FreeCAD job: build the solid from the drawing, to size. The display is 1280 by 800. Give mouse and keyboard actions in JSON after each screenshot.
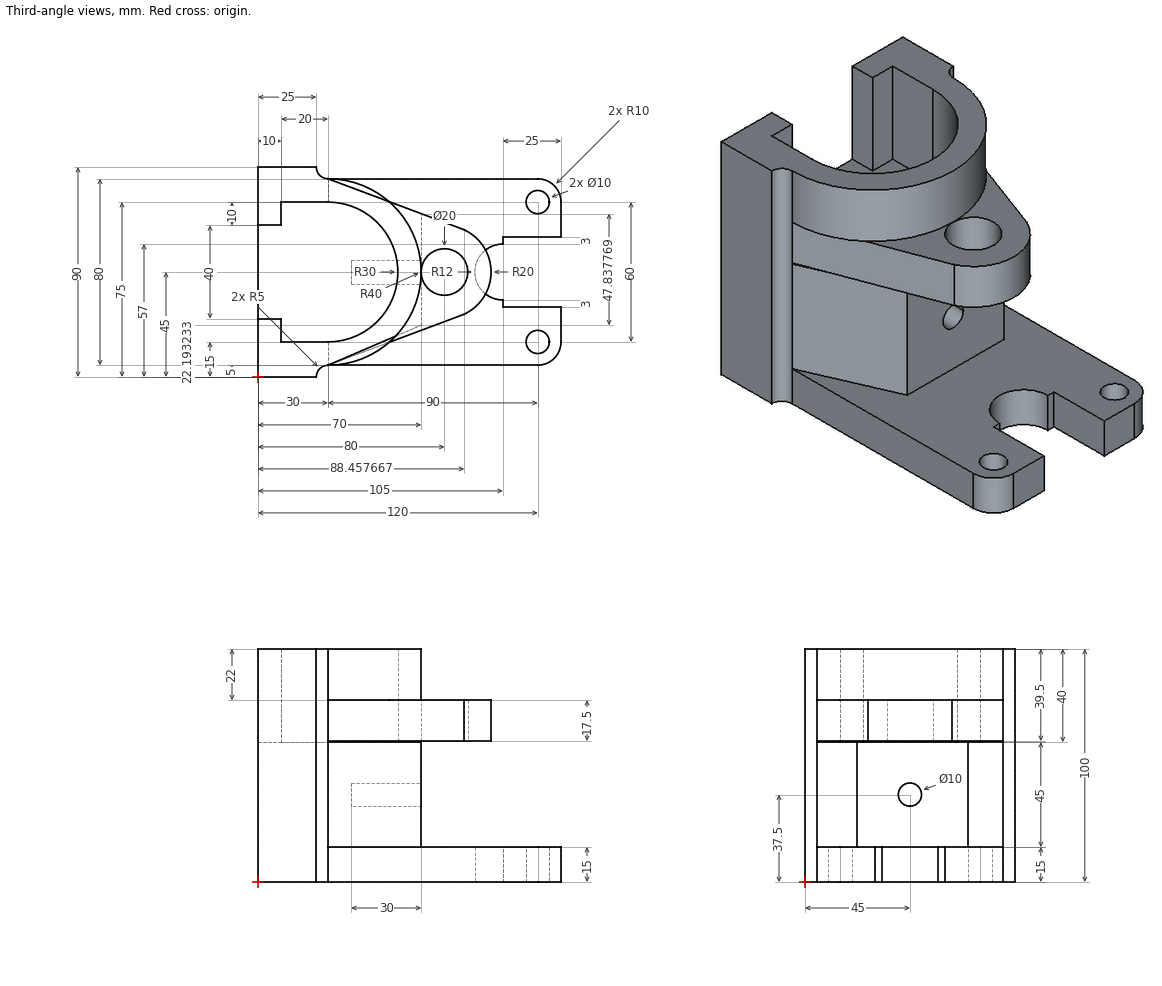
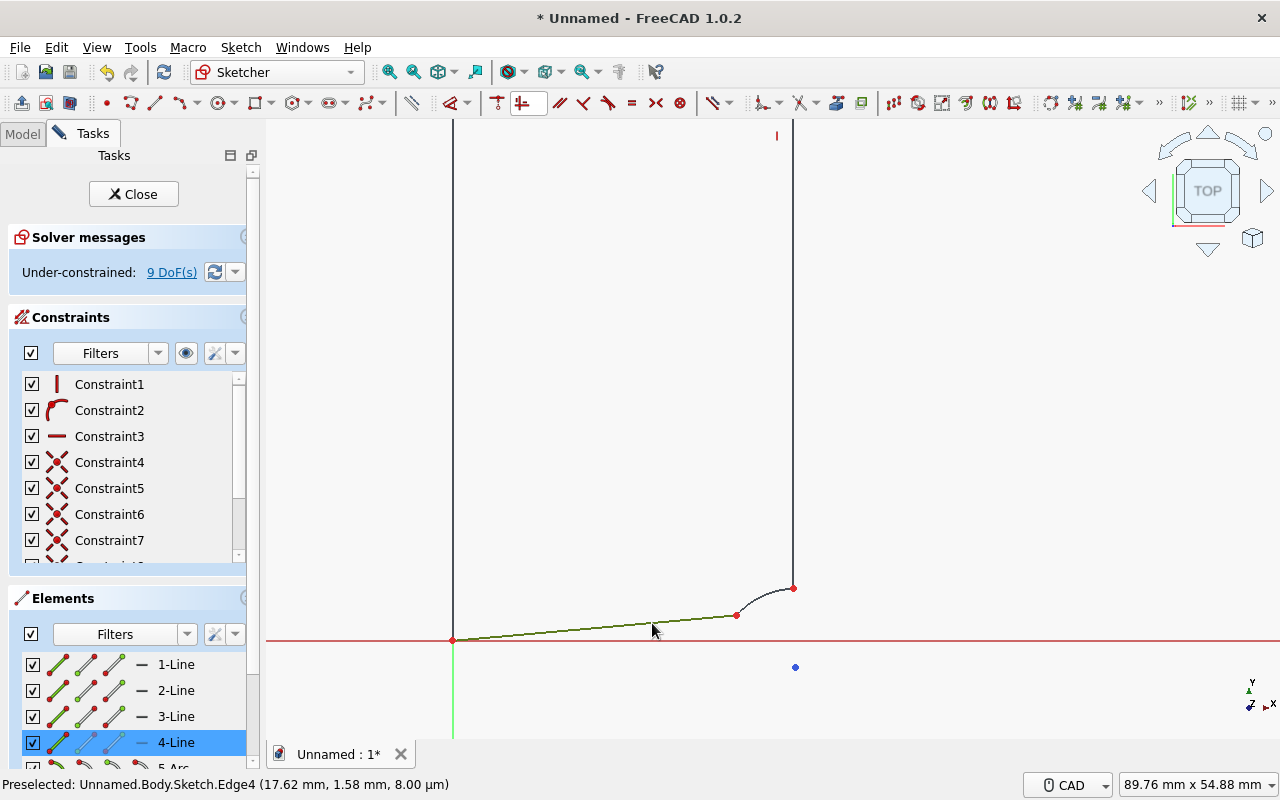
{"action": "left_click", "coordinate": [542, 104]}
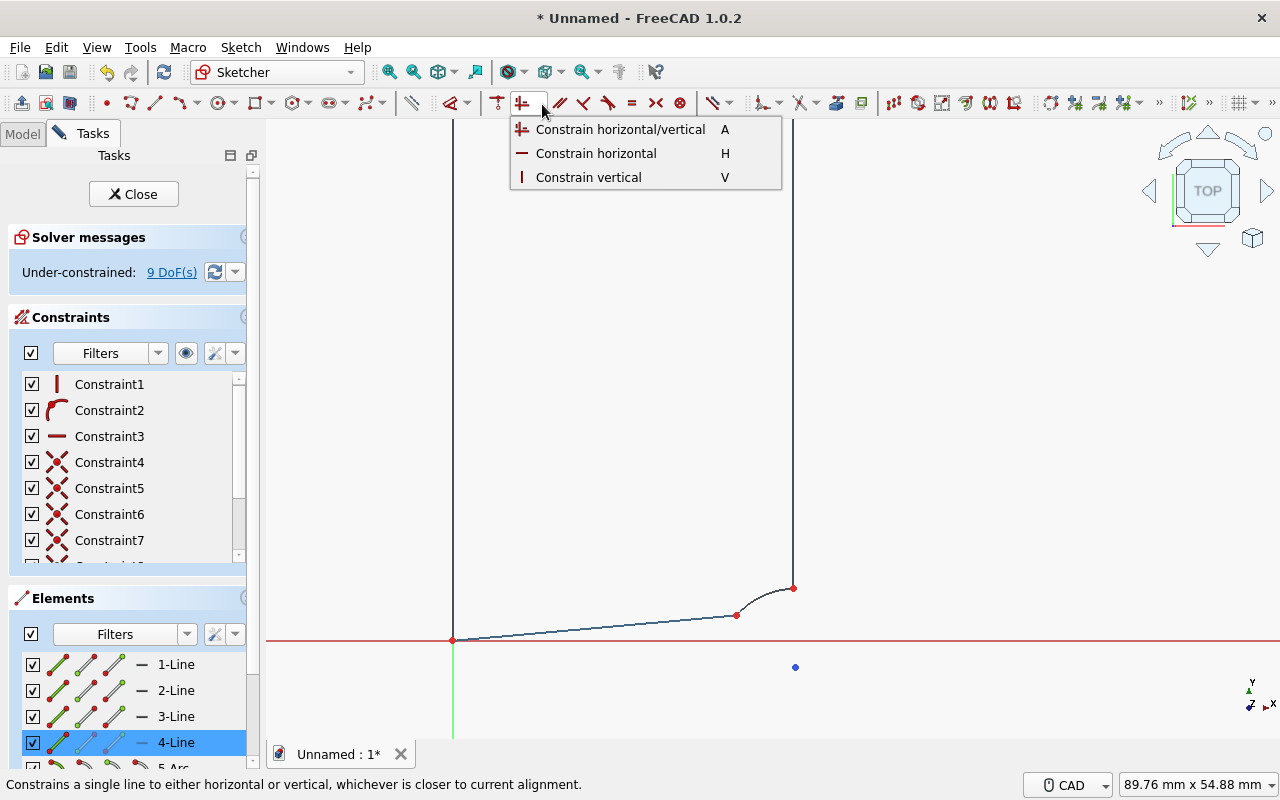
{"action": "left_click", "coordinate": [646, 153]}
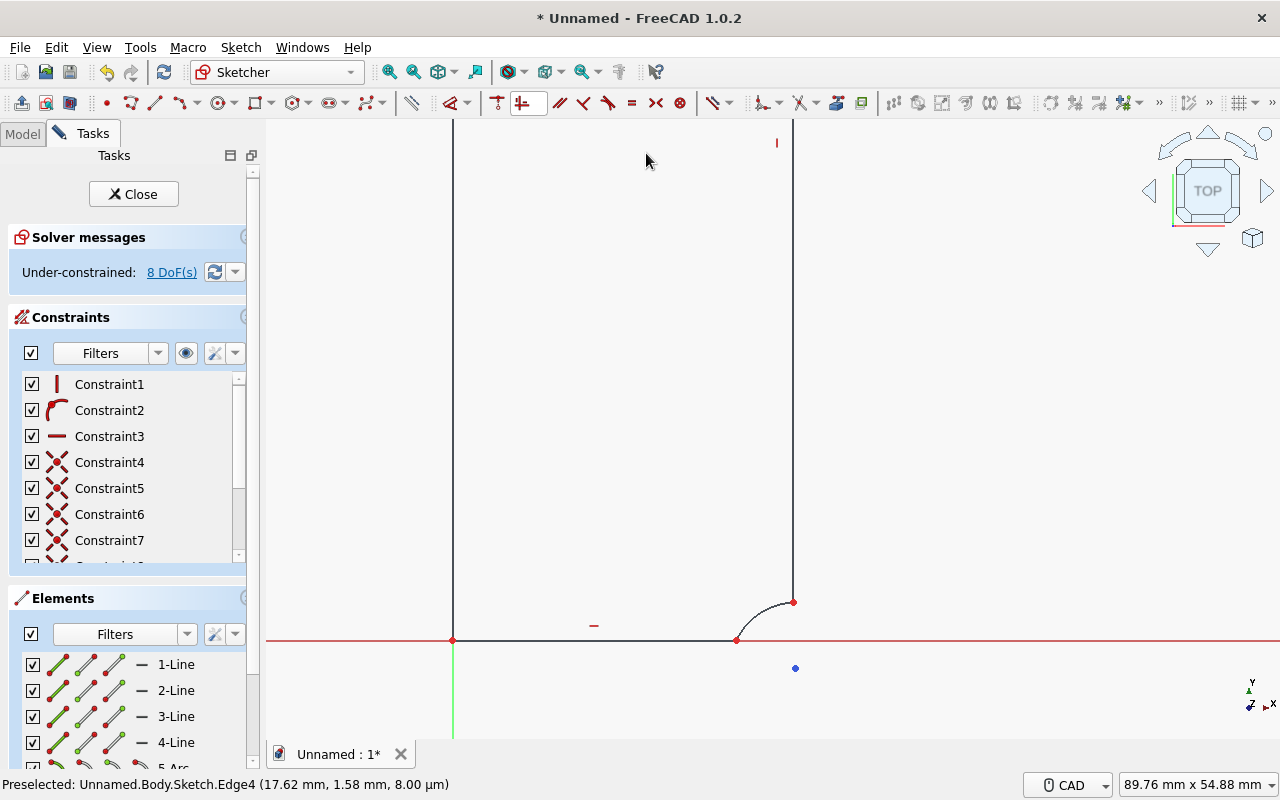
{"action": "scroll", "coordinate": [752, 602], "scroll_direction": "down", "scroll_amount": 5}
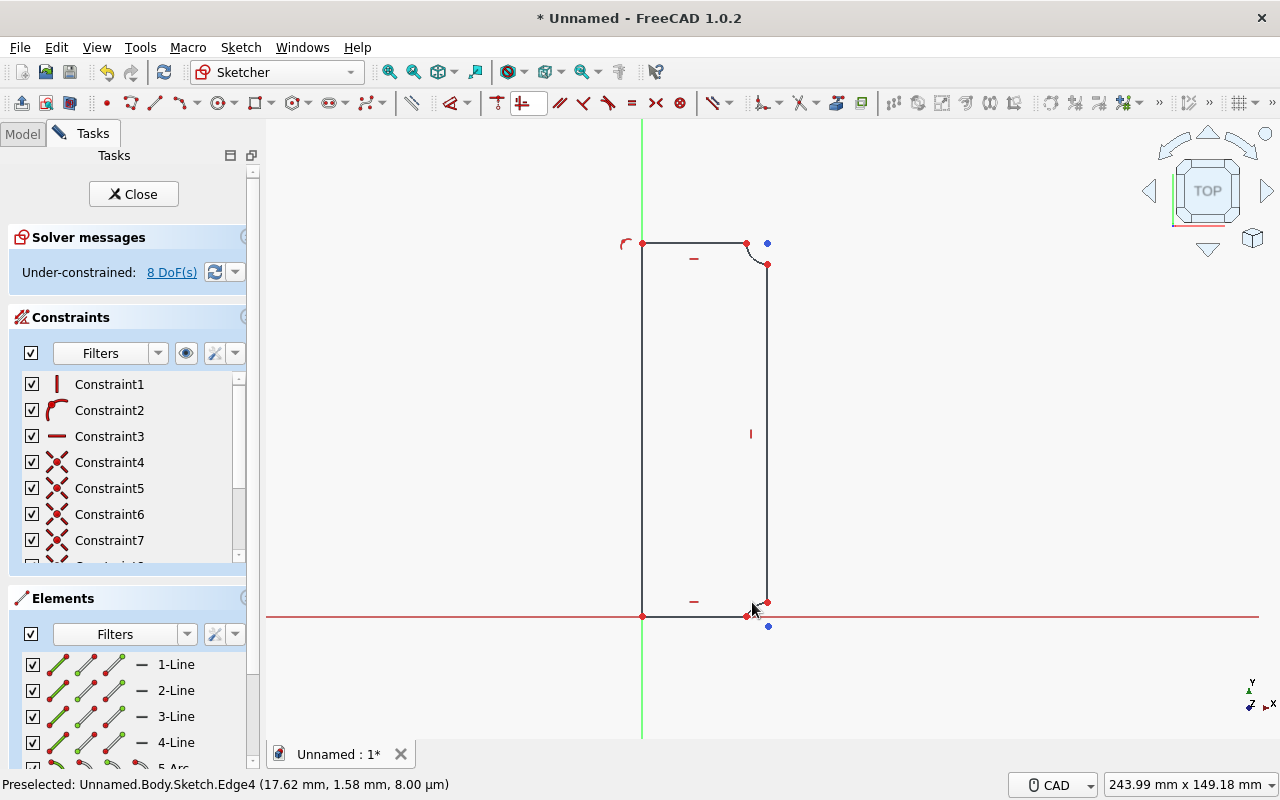
{"action": "scroll", "coordinate": [749, 253], "scroll_direction": "up", "scroll_amount": 2}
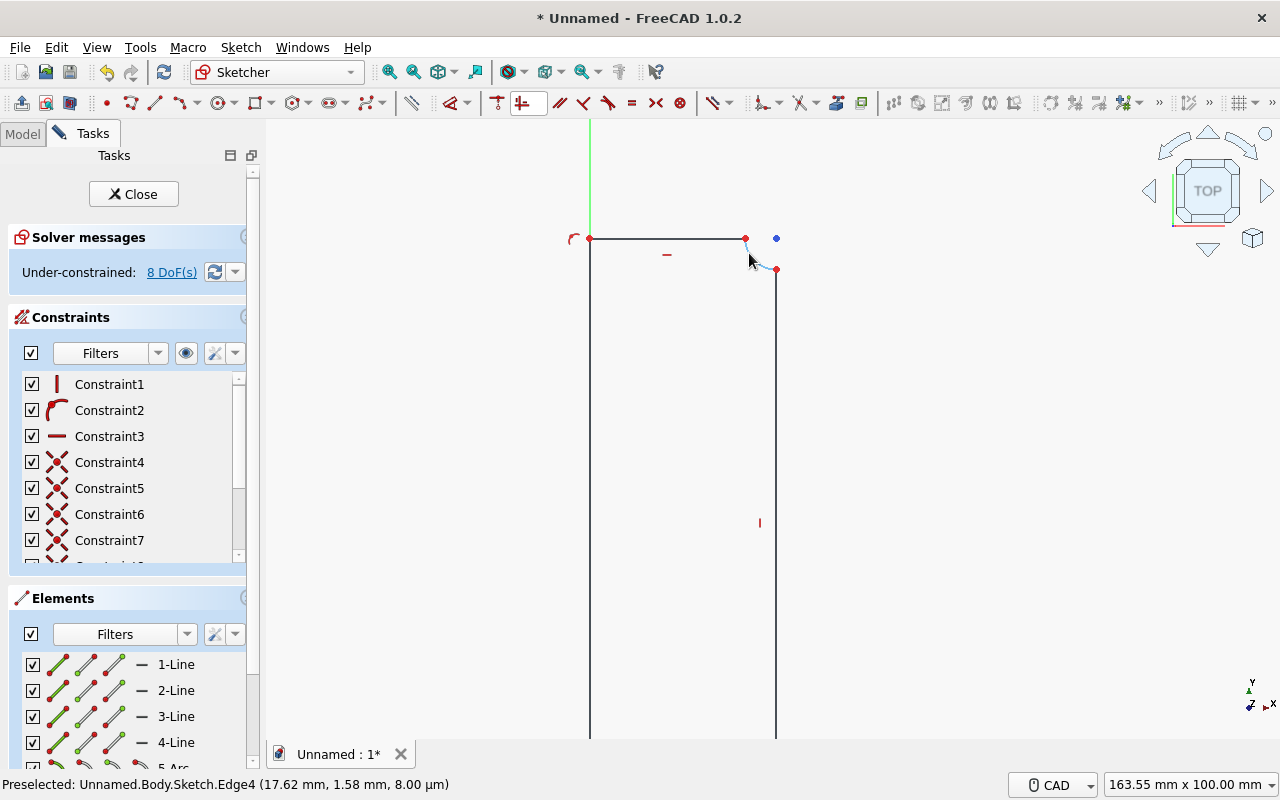
{"action": "left_click", "coordinate": [749, 253]}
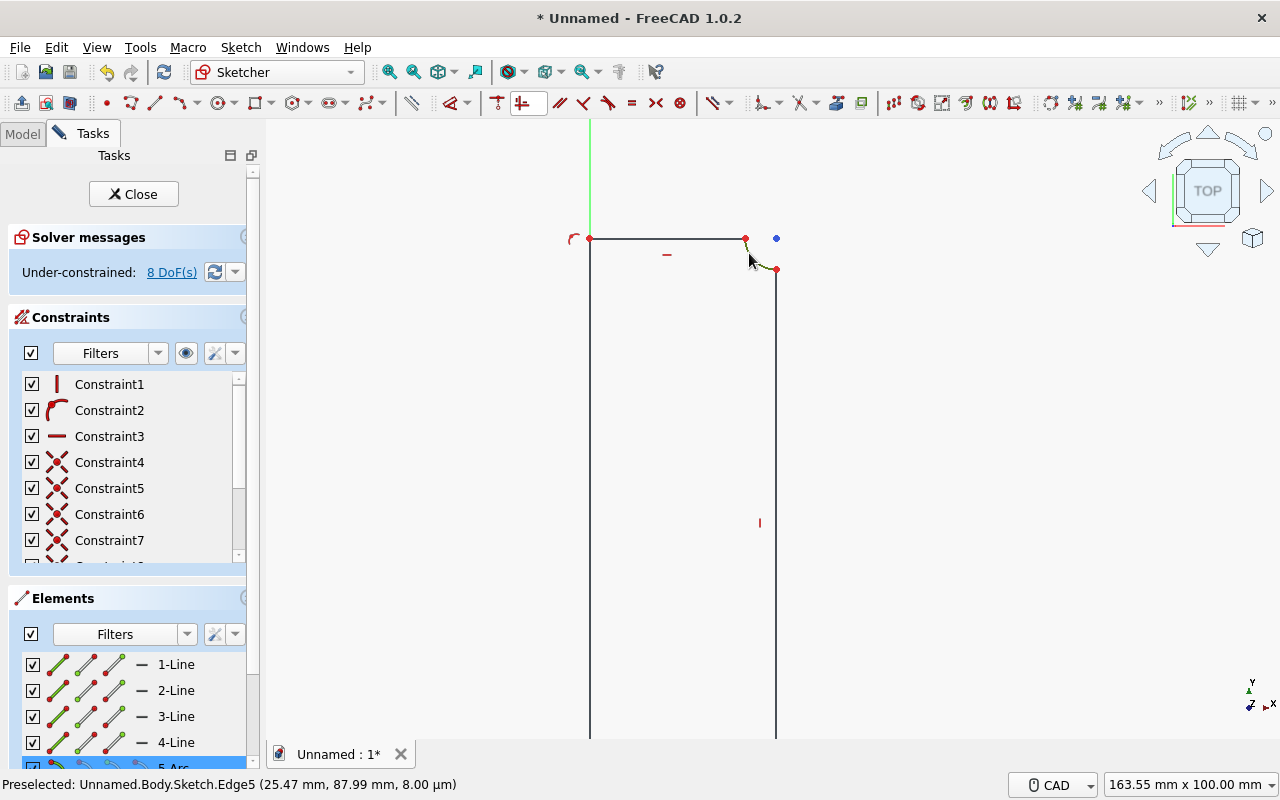
{"action": "scroll", "coordinate": [749, 251], "scroll_direction": "down", "scroll_amount": 2}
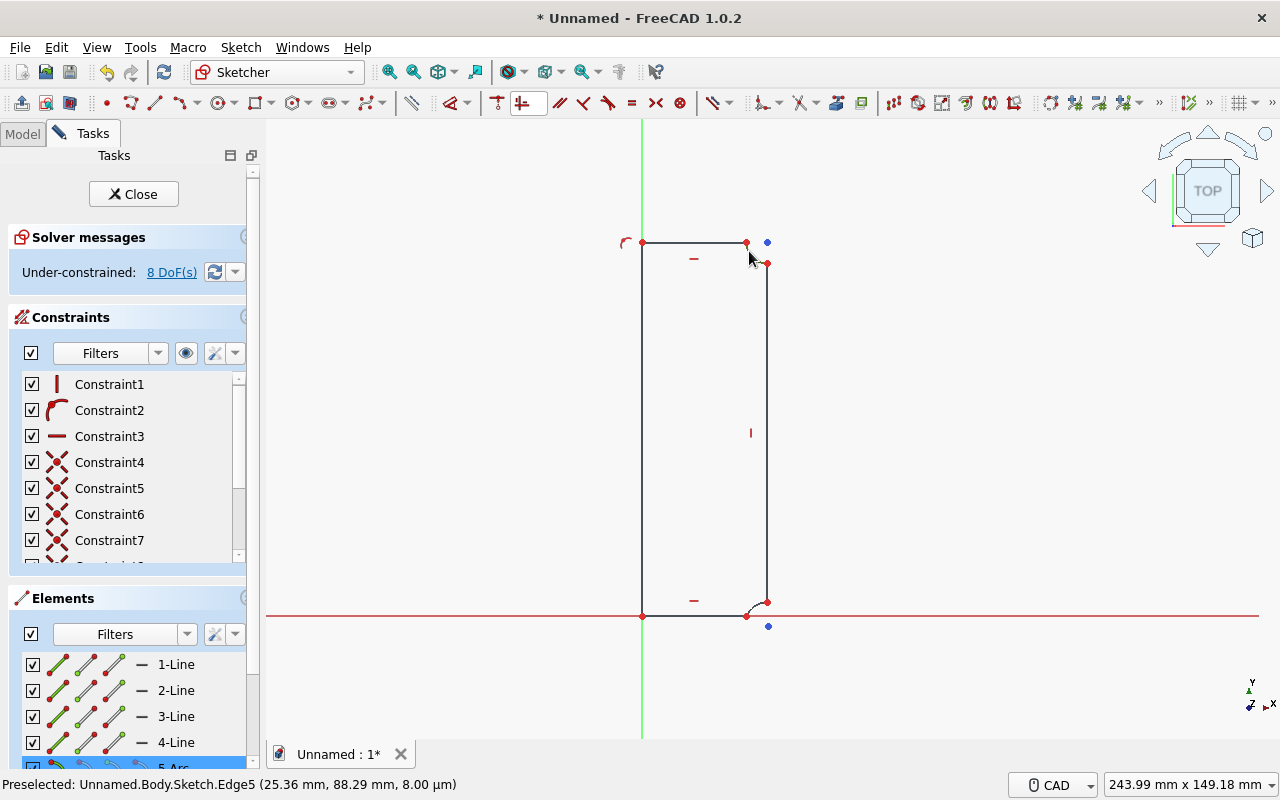
{"action": "scroll", "coordinate": [760, 604], "scroll_direction": "up", "scroll_amount": 3}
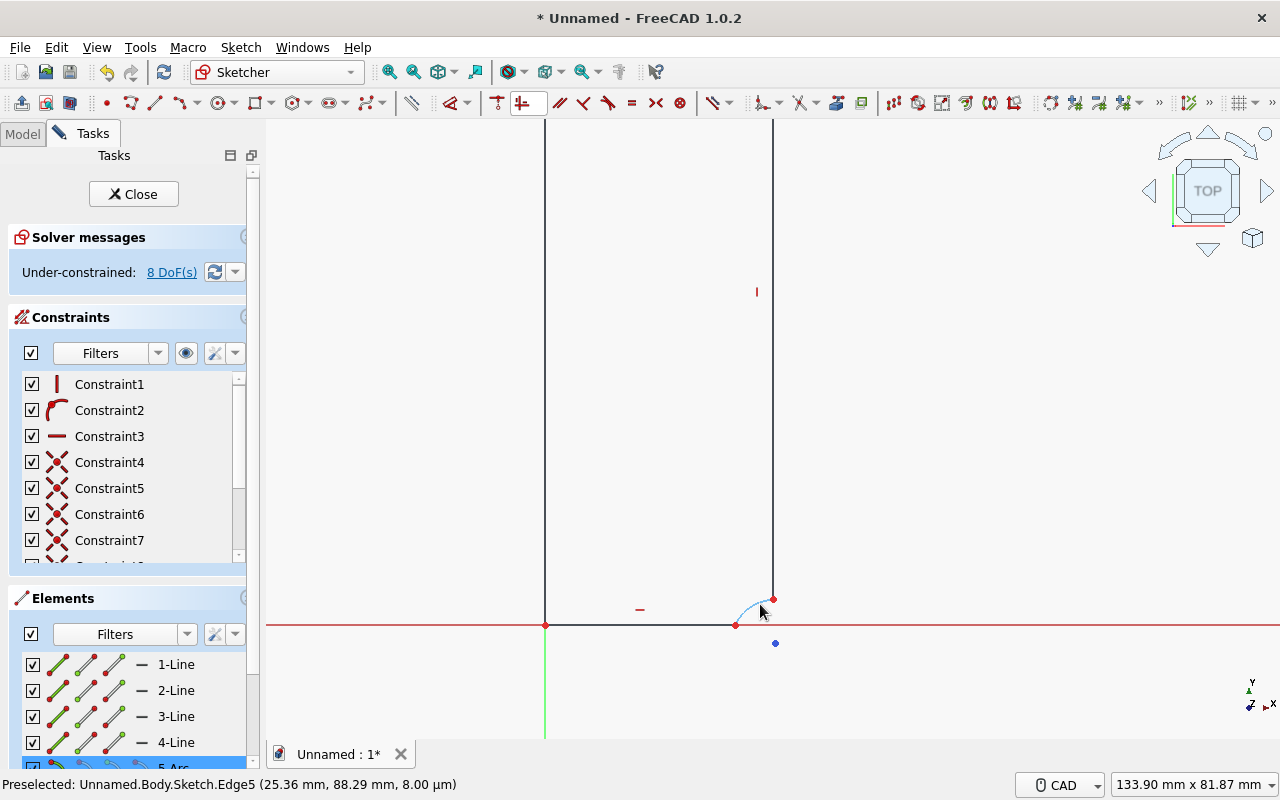
{"action": "left_click", "coordinate": [759, 603]}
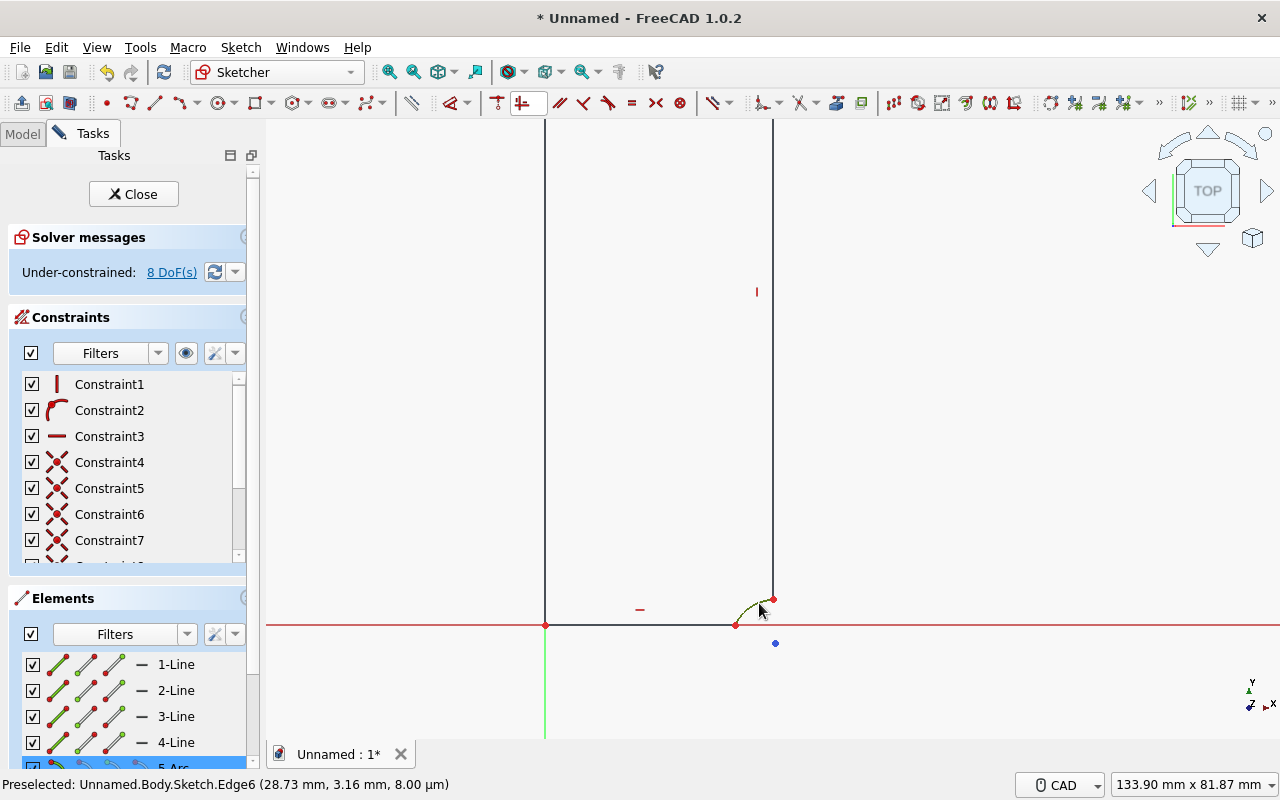
{"action": "left_click", "coordinate": [632, 104]}